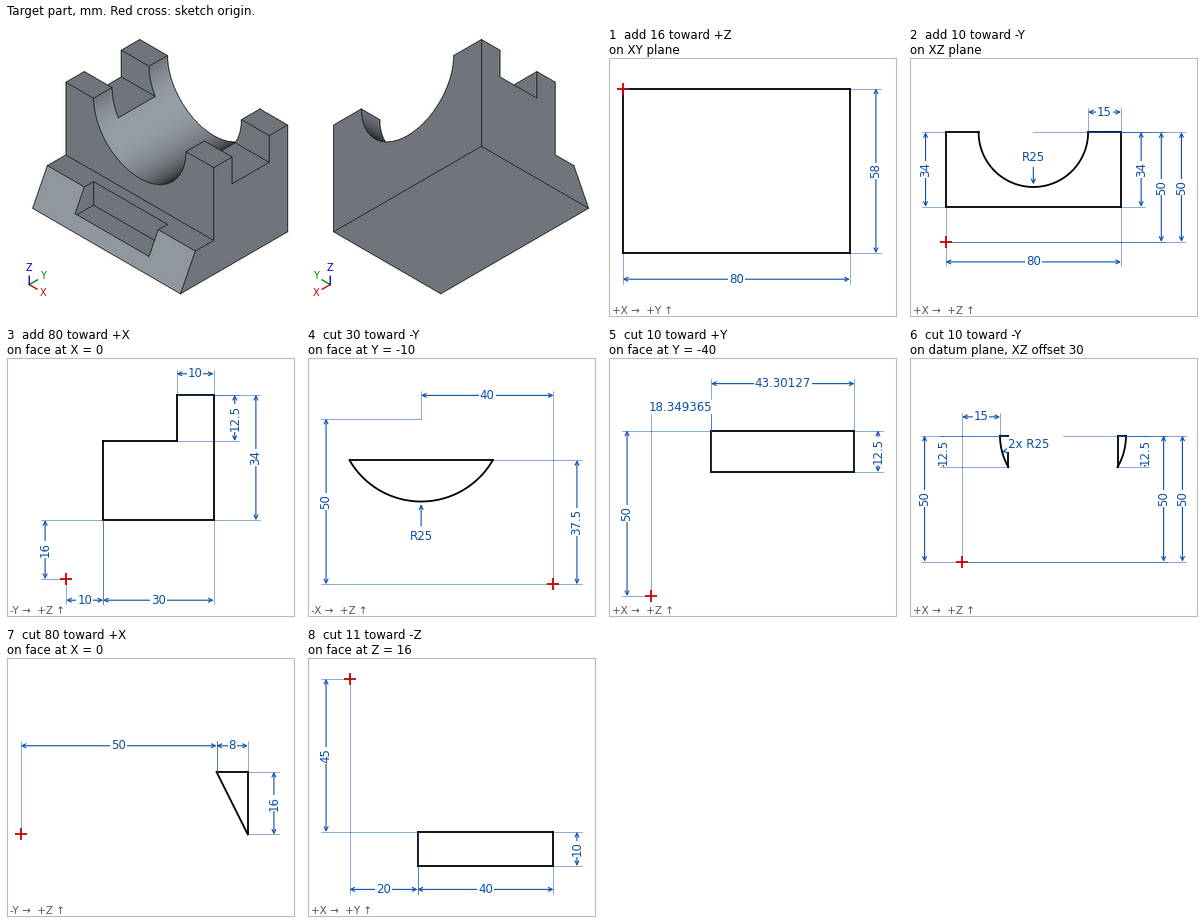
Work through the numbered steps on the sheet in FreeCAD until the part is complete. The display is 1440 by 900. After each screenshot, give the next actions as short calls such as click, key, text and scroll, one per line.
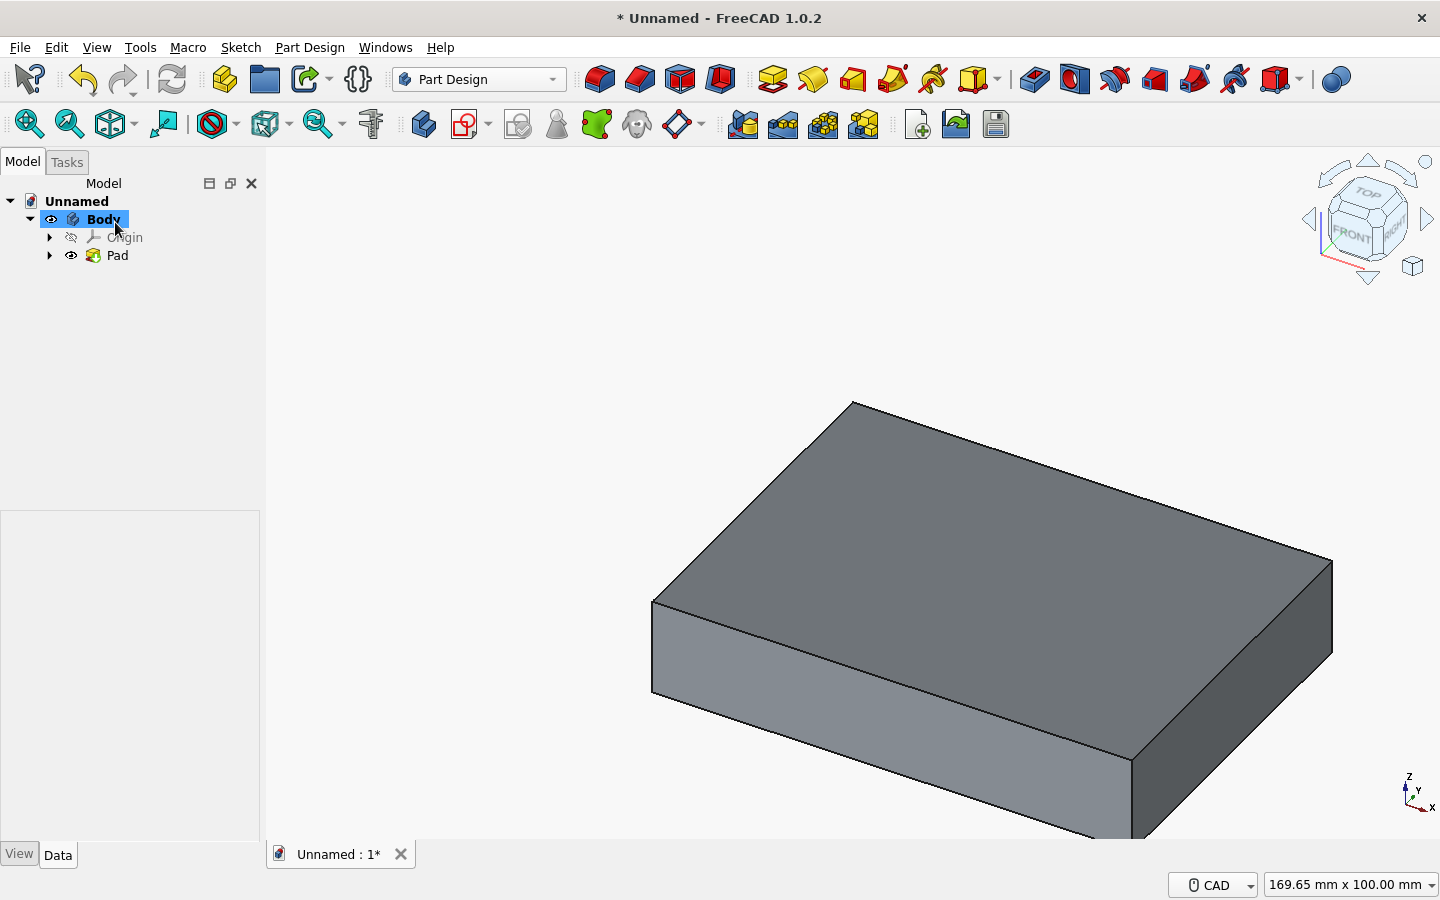
click(30, 124)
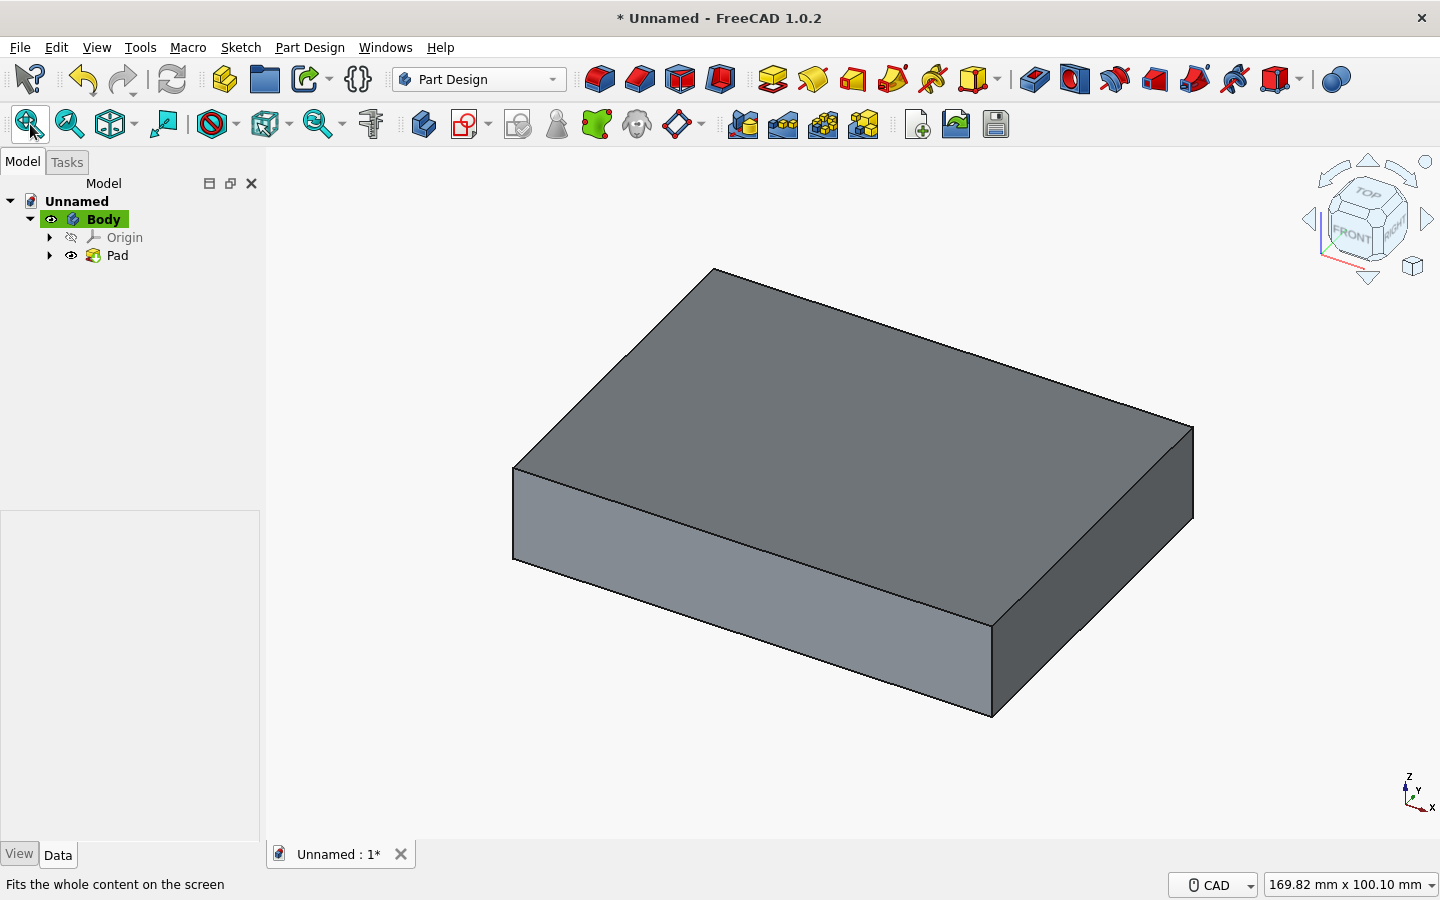
click(464, 124)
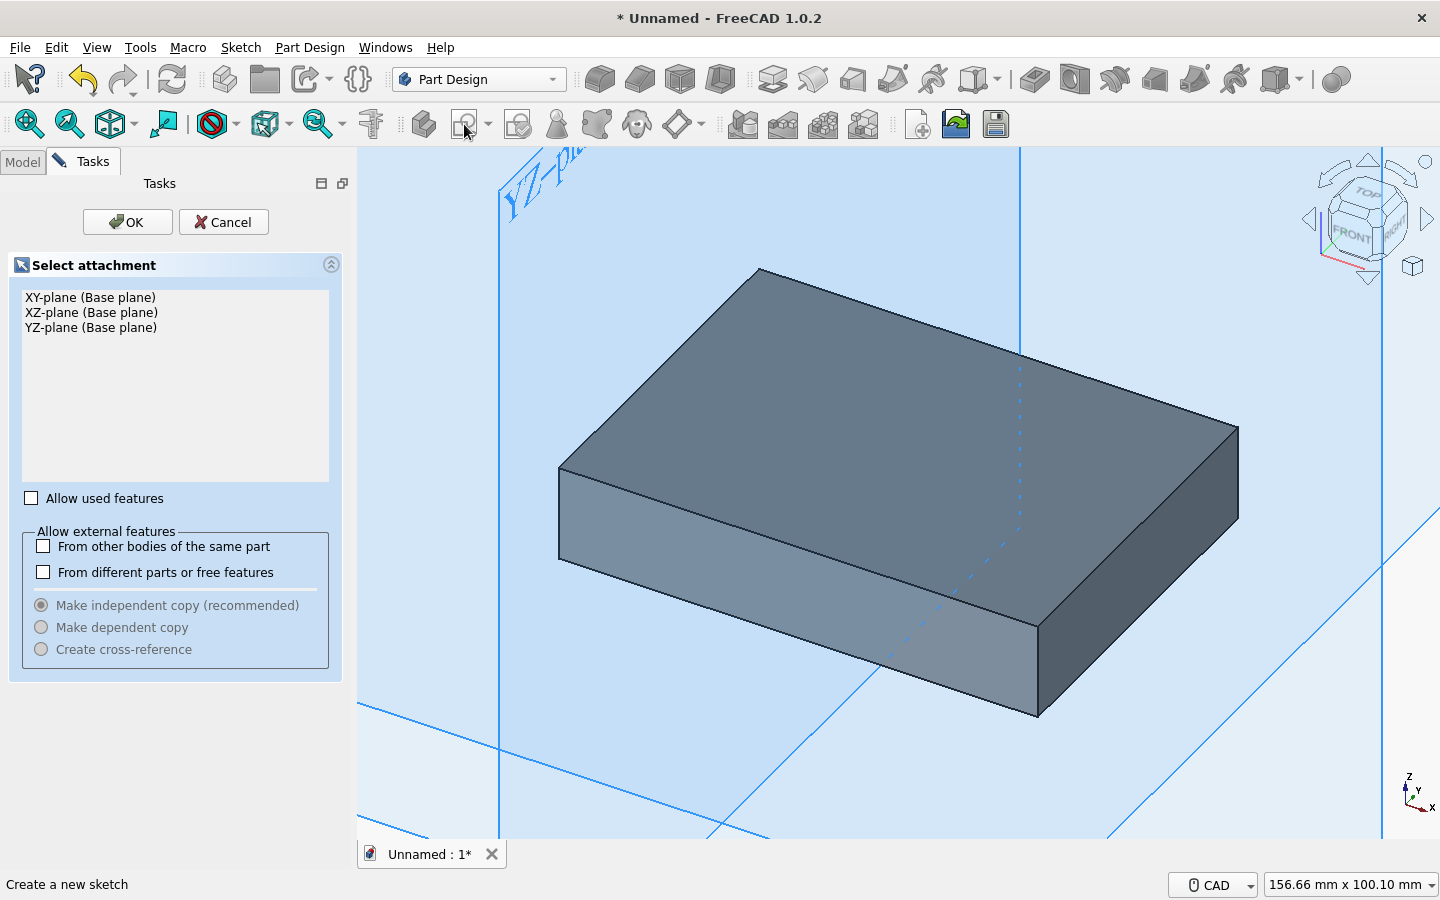
click(82, 312)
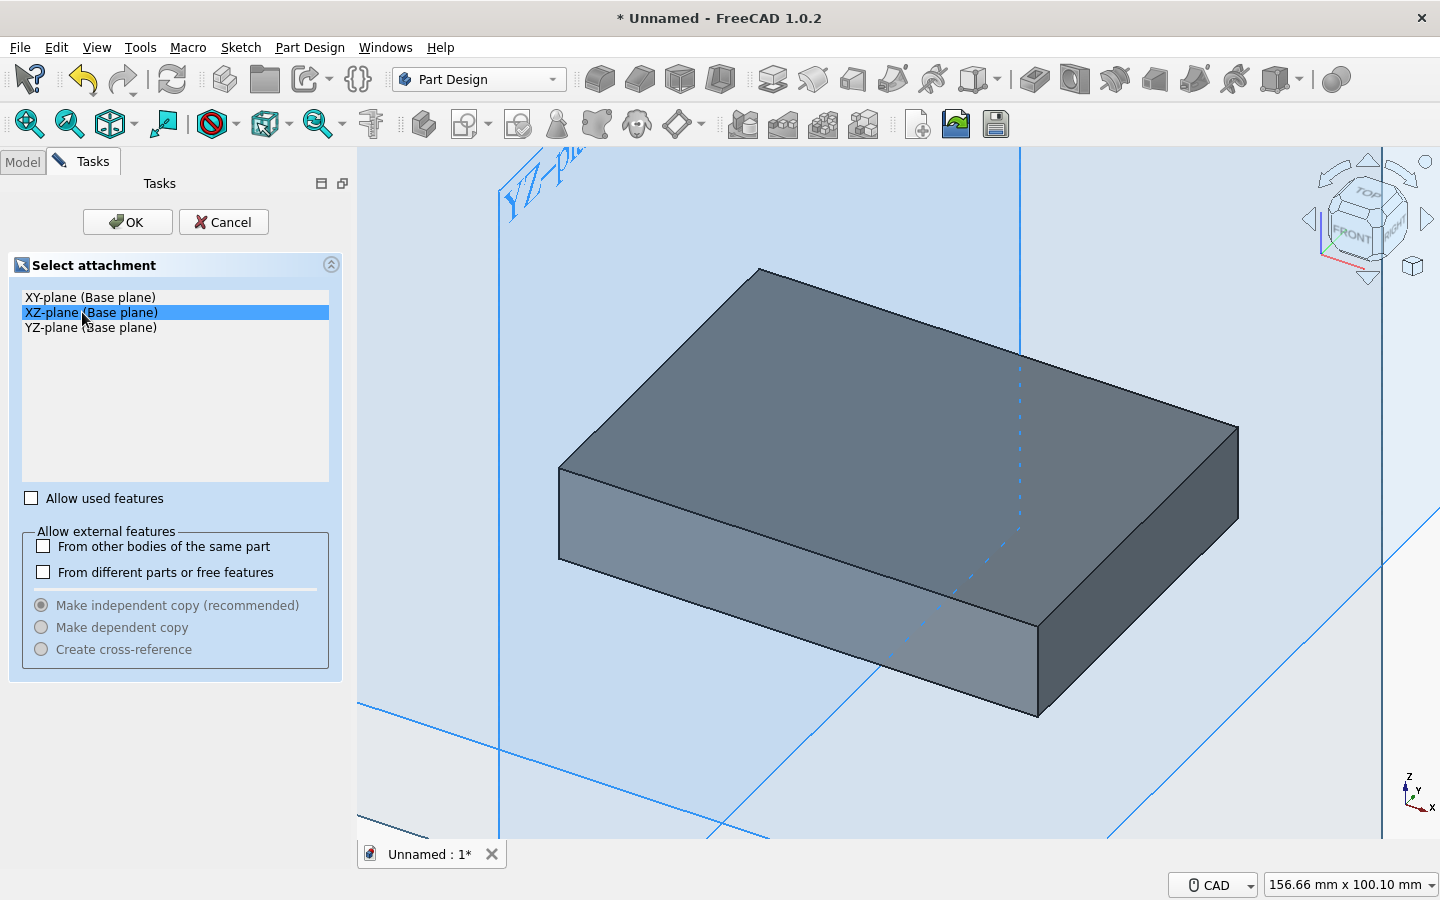
click(128, 222)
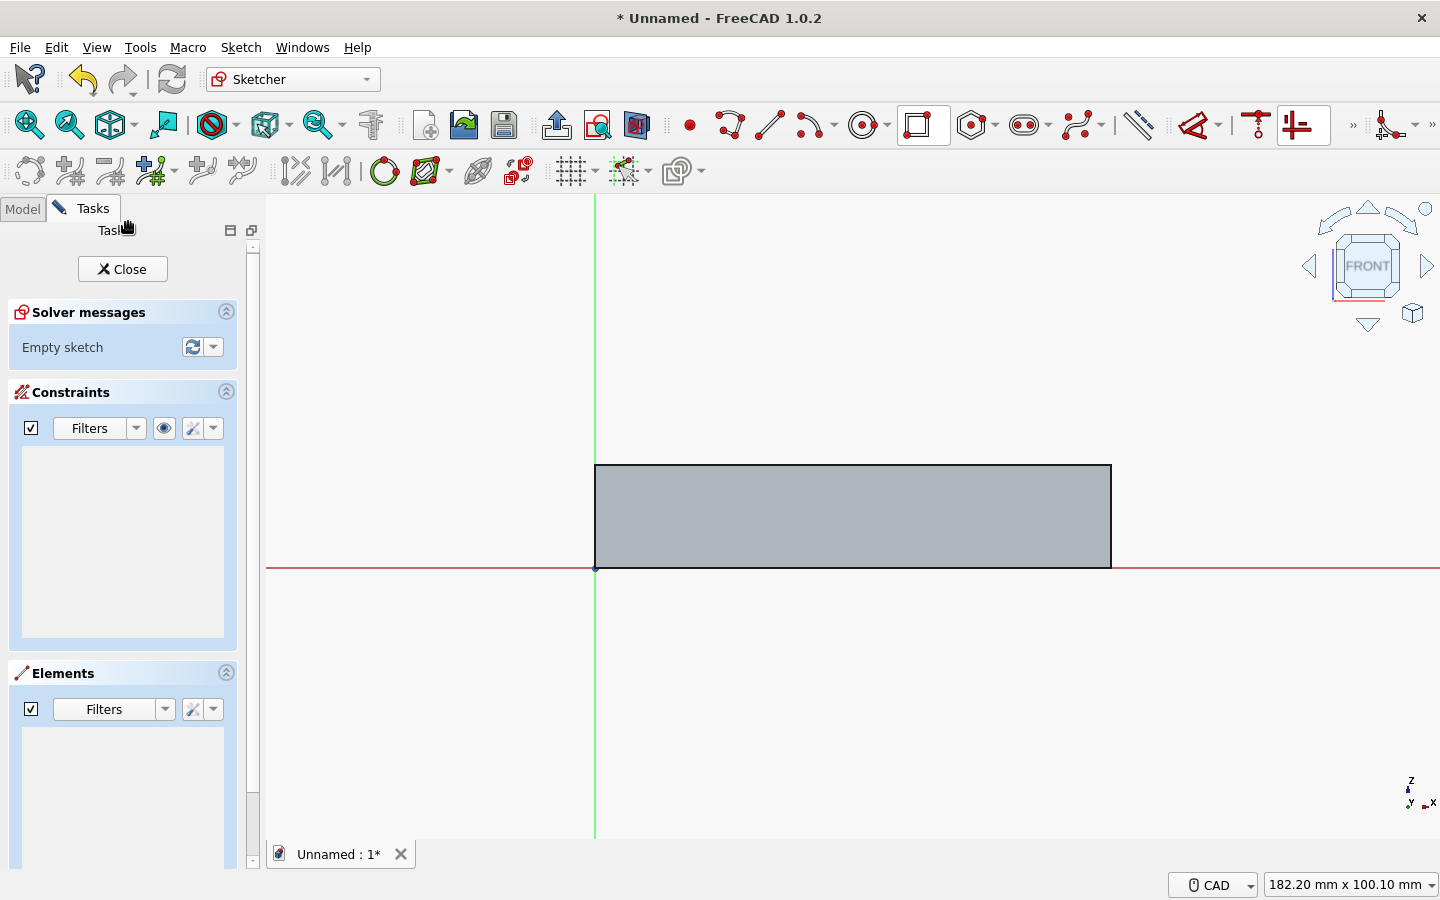
click(638, 126)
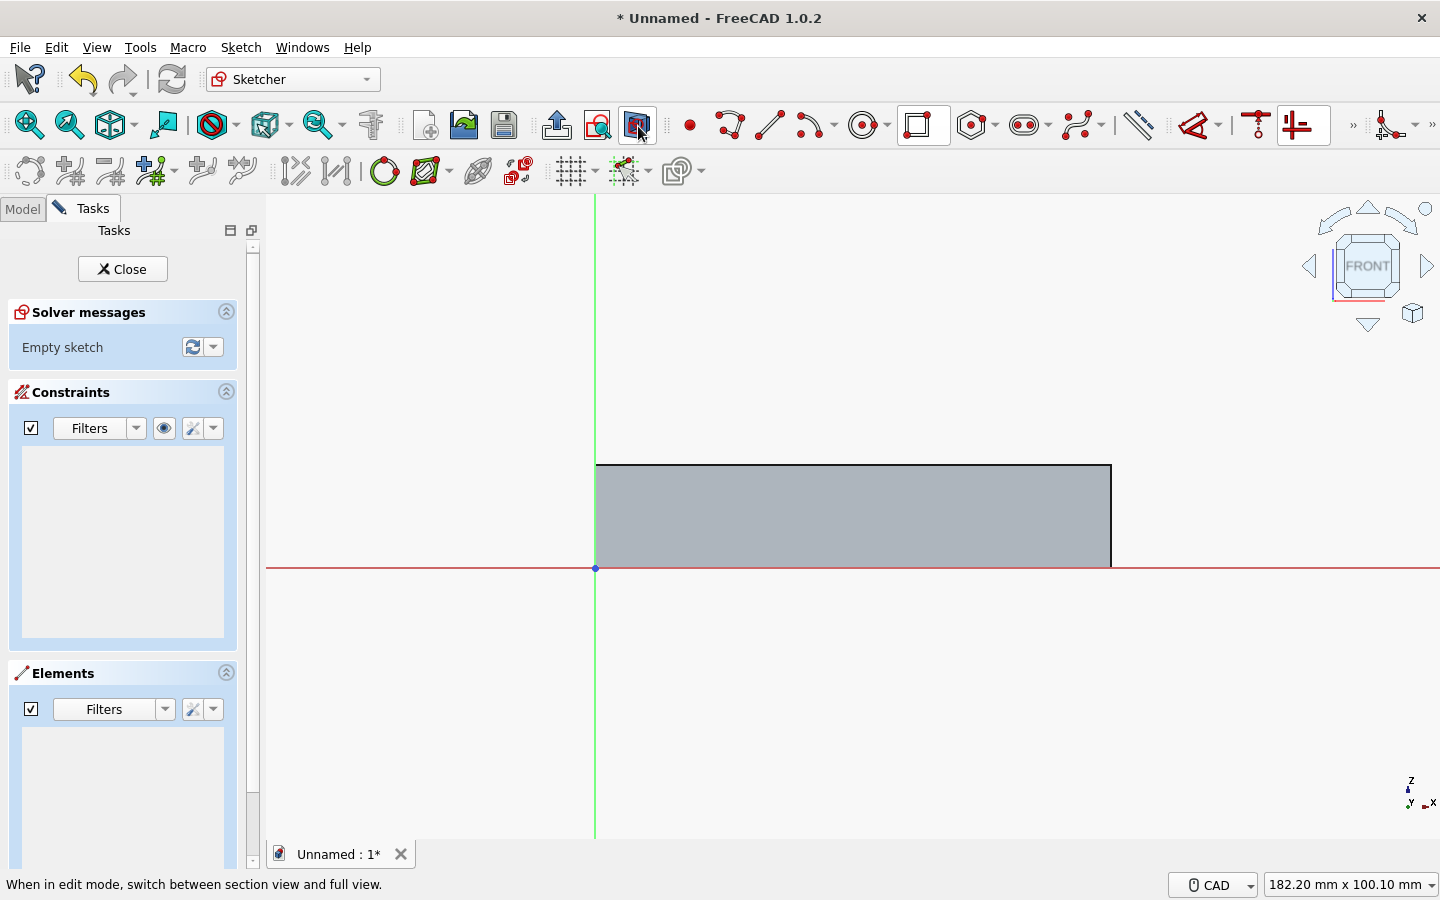
scroll(1162, 222, up, 1)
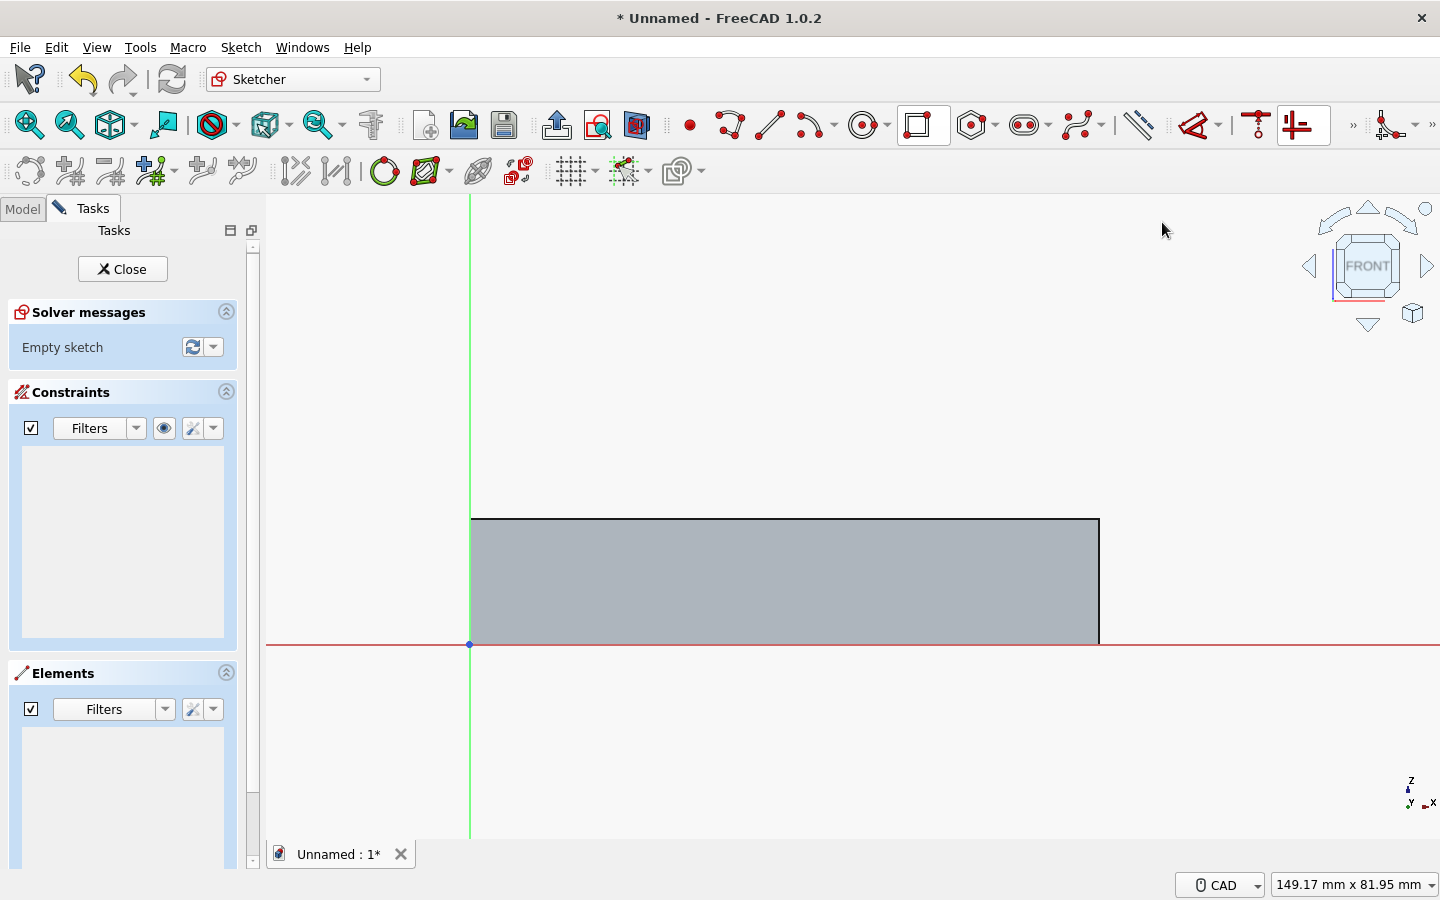
click(730, 126)